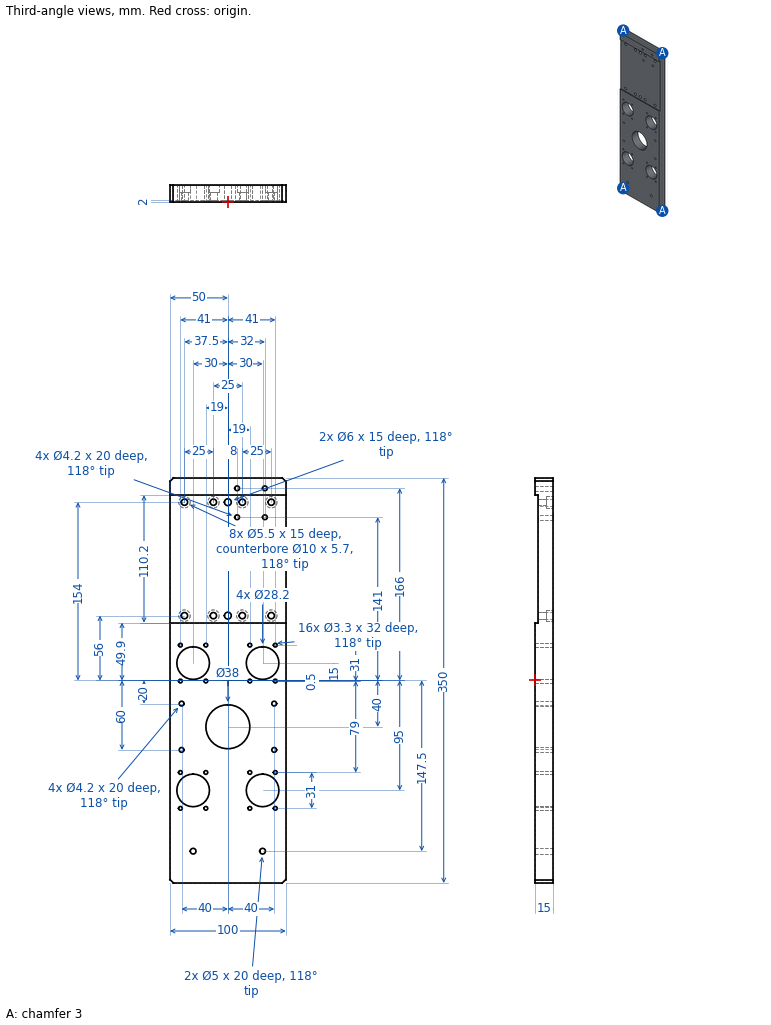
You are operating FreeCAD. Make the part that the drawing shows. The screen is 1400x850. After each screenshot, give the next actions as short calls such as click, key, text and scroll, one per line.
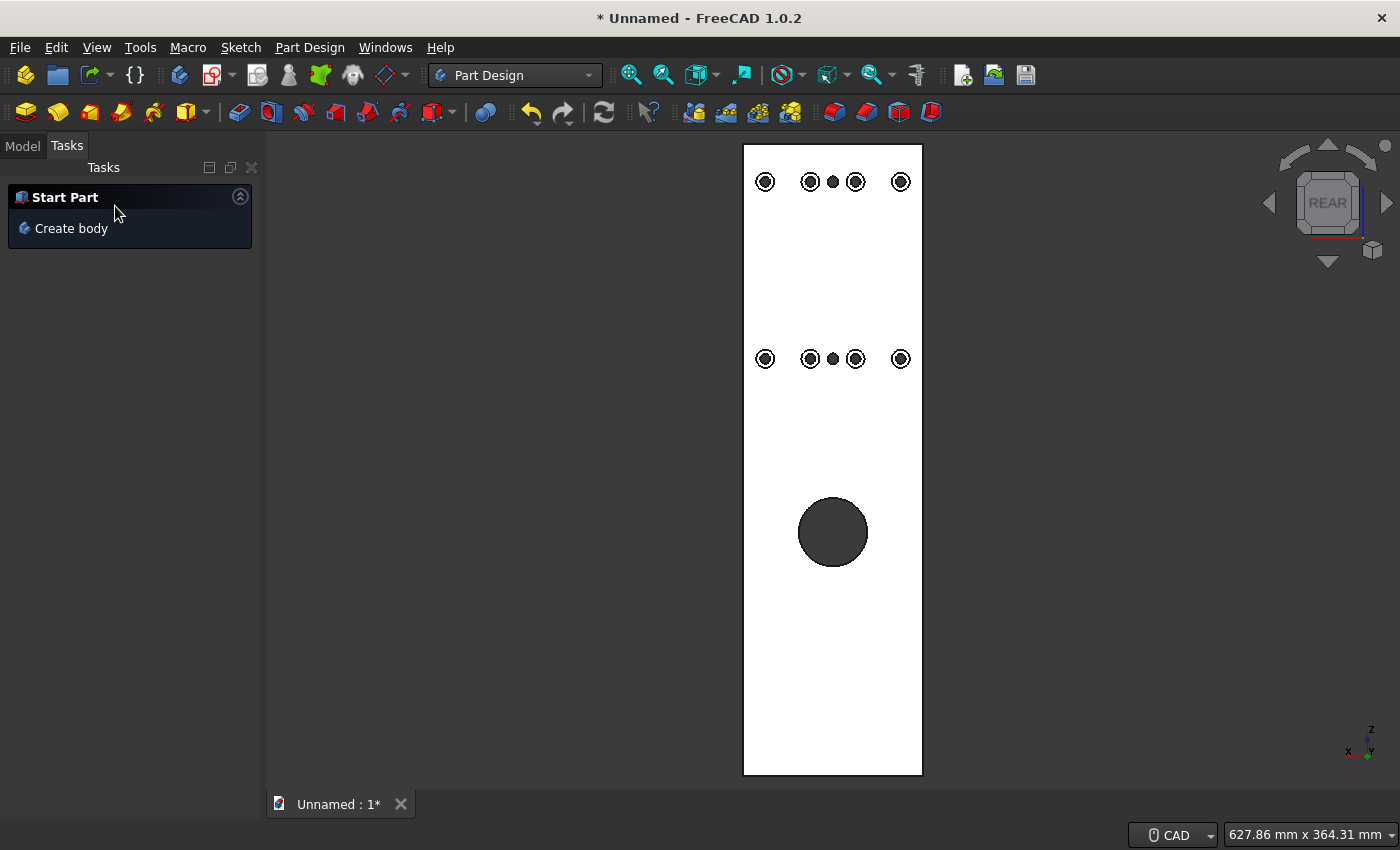
key(0)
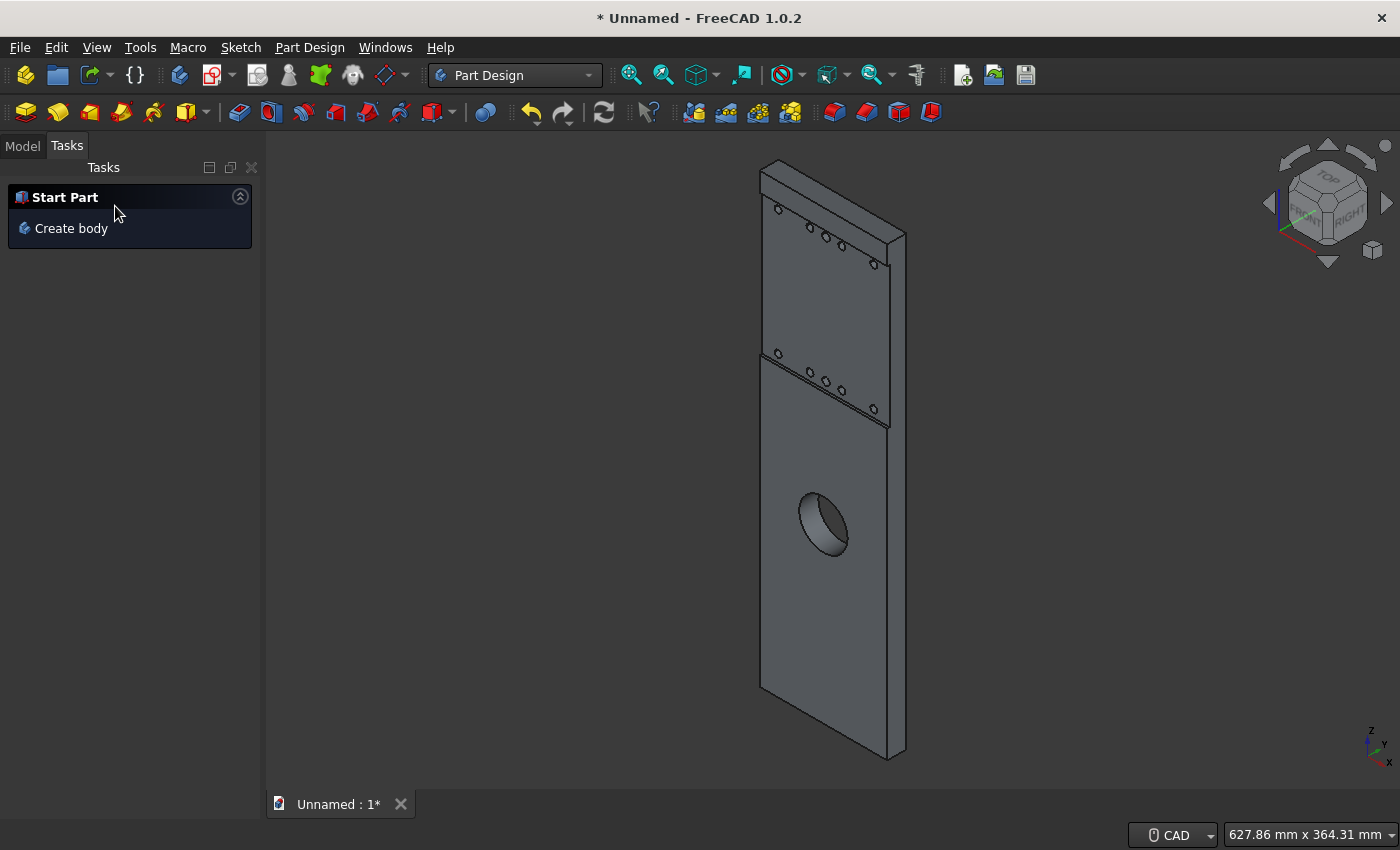
click(897, 238)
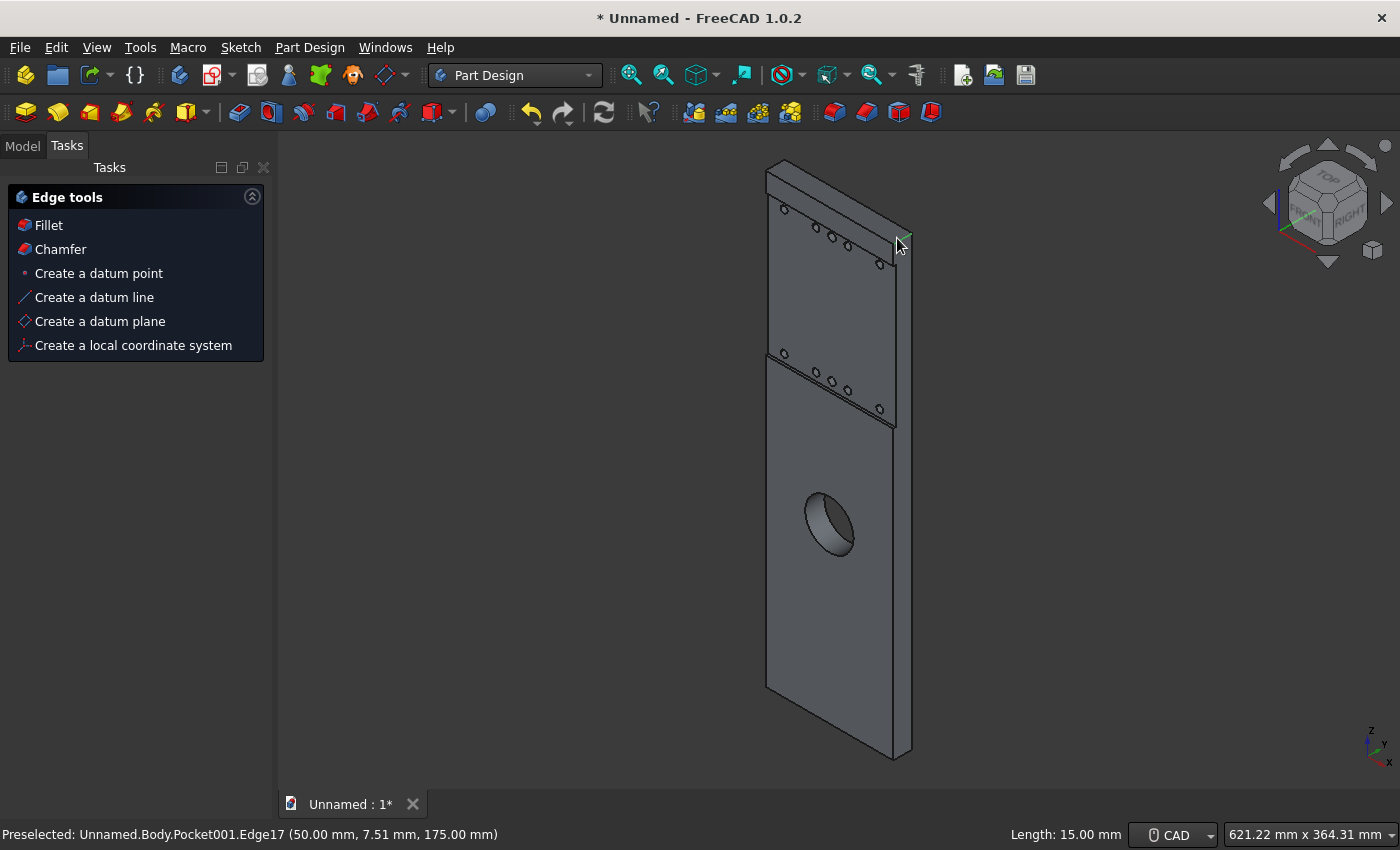
key(2)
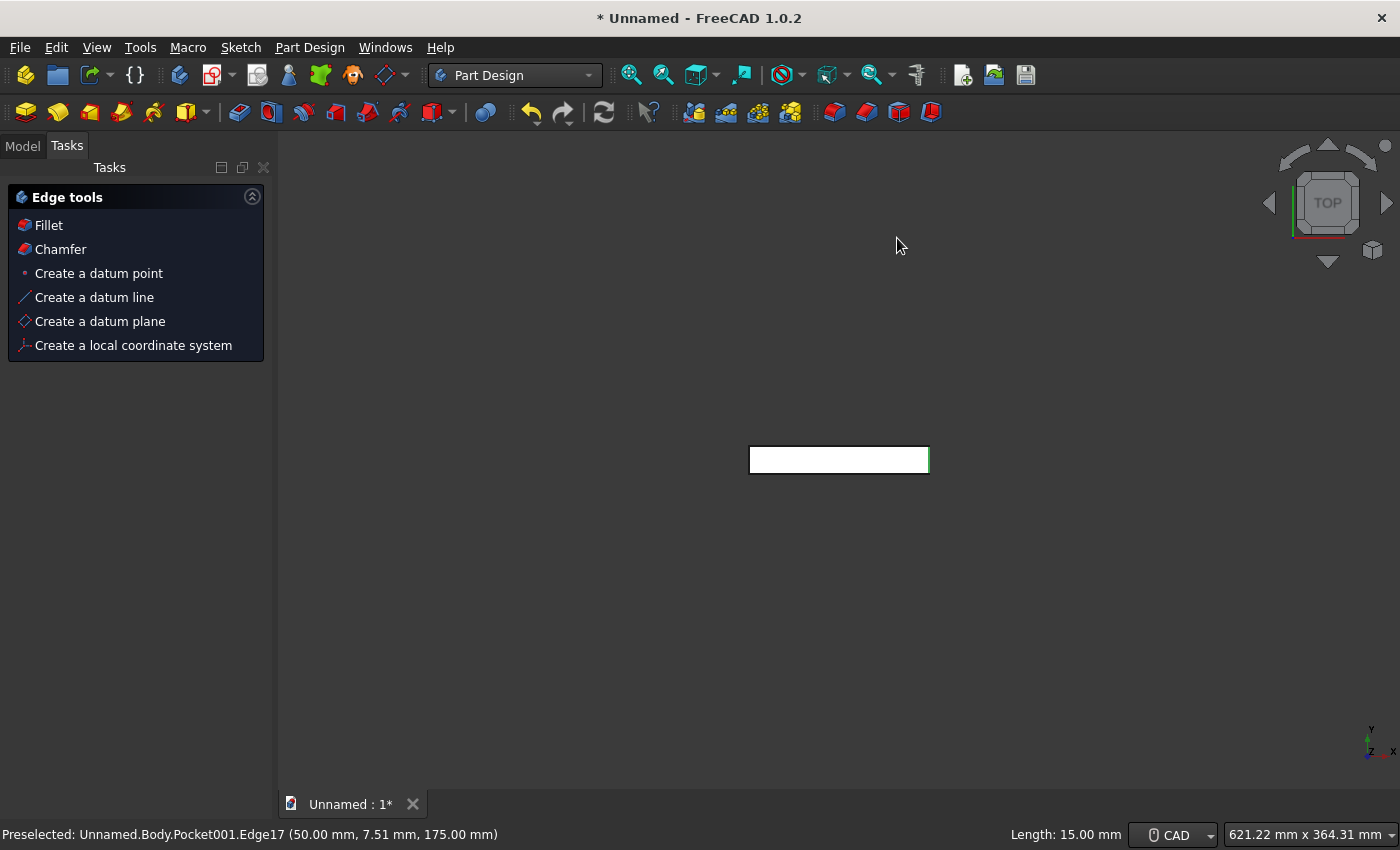
click(632, 76)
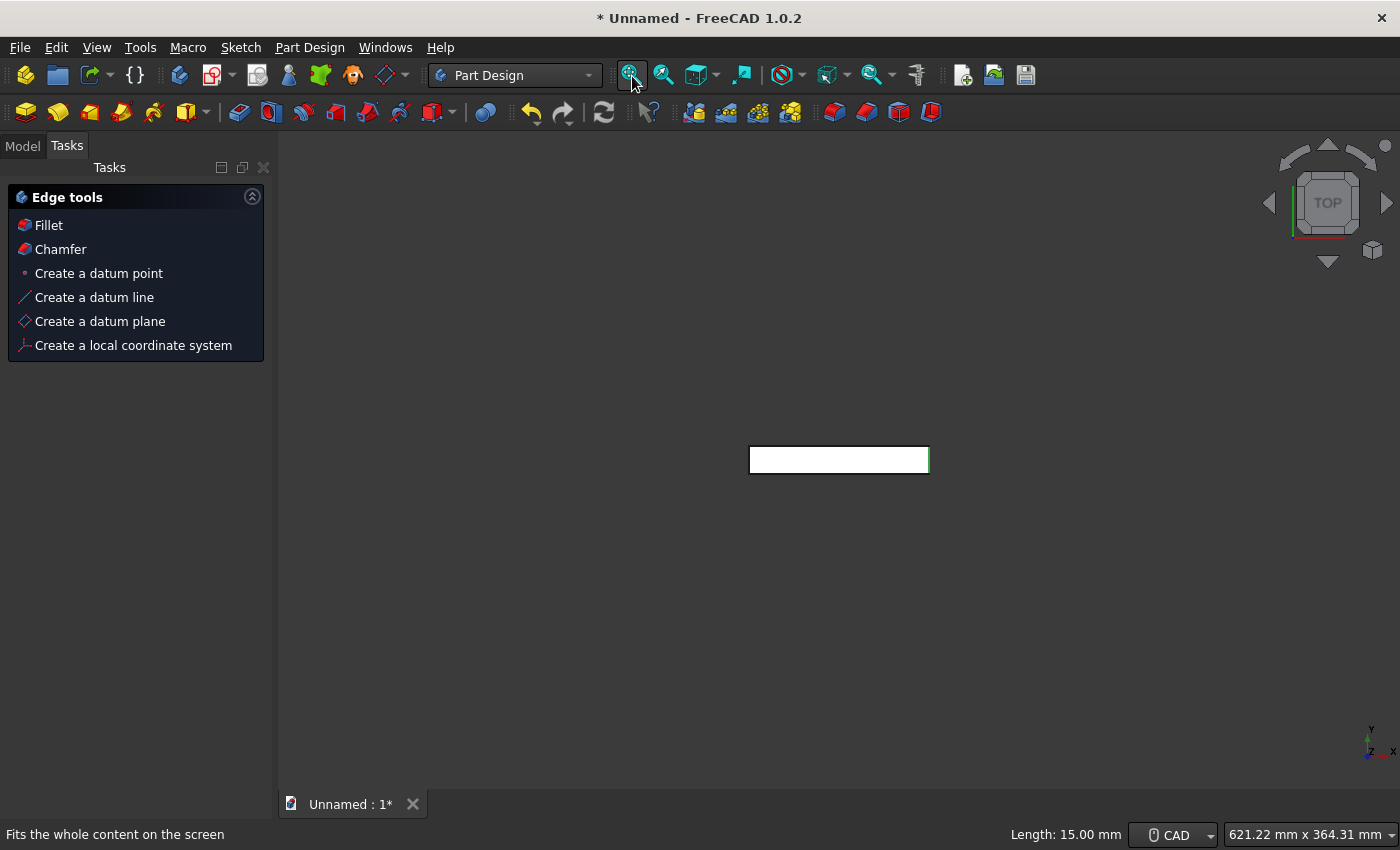
click(749, 459, ctrl)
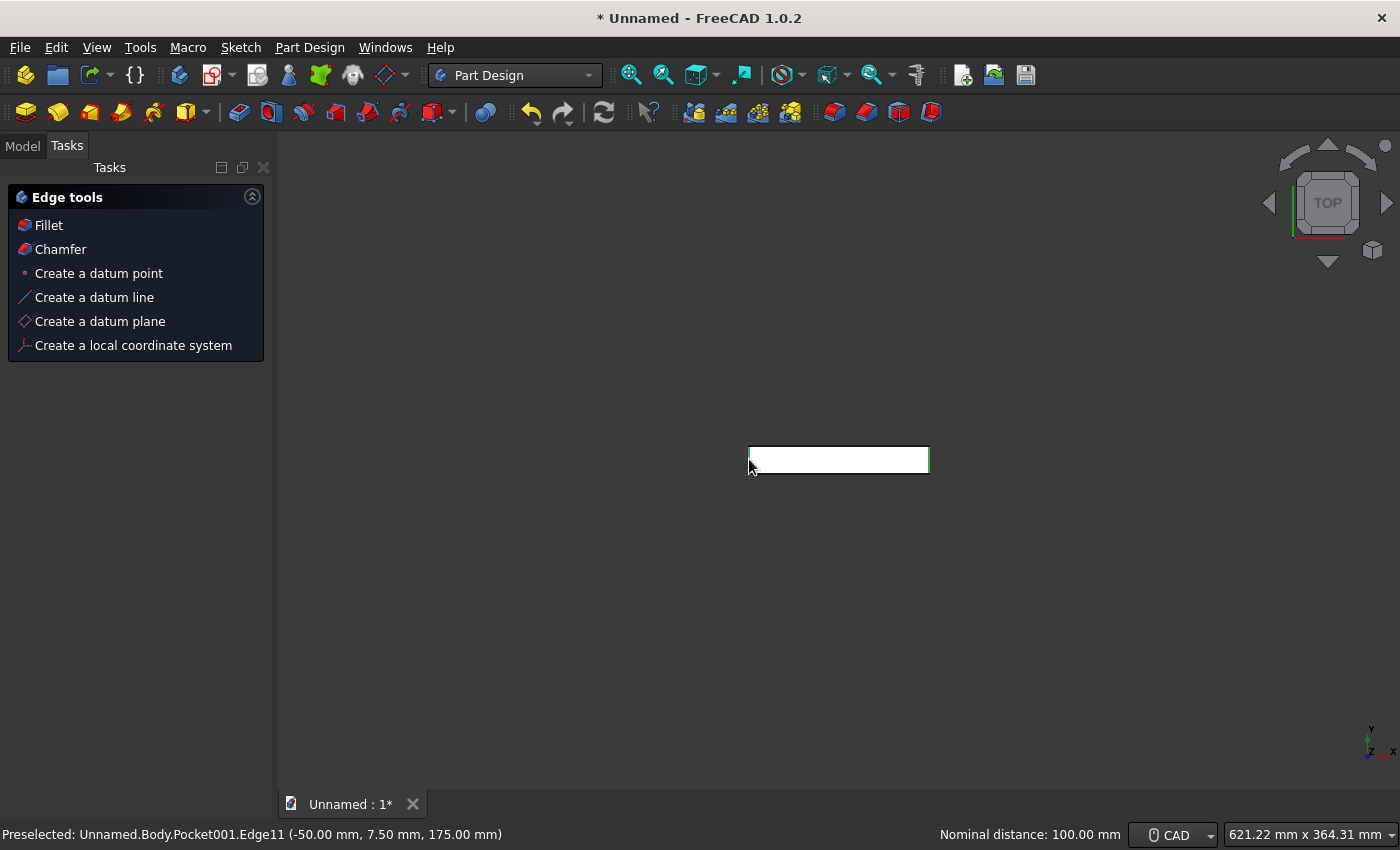
key(1)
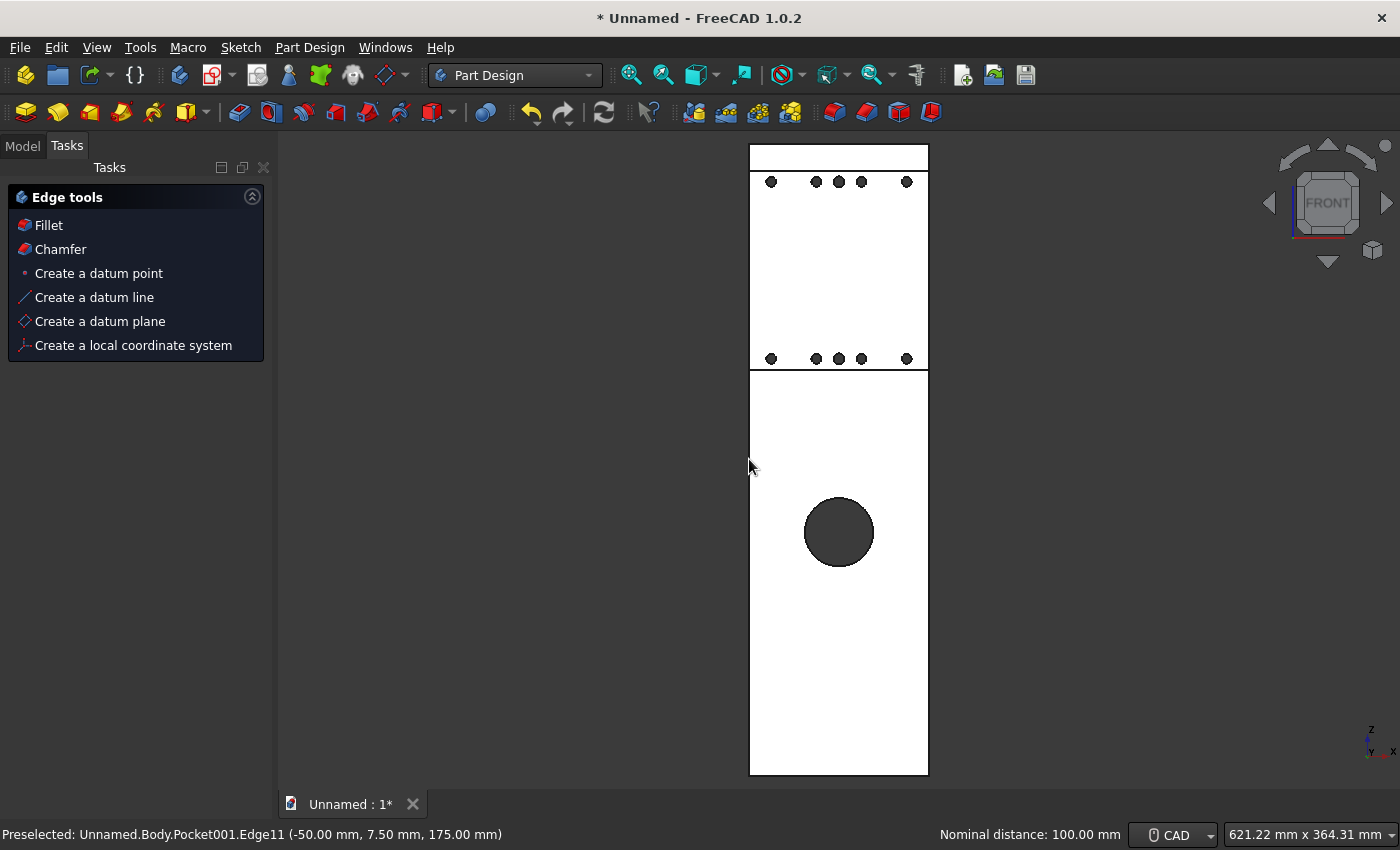
key(3)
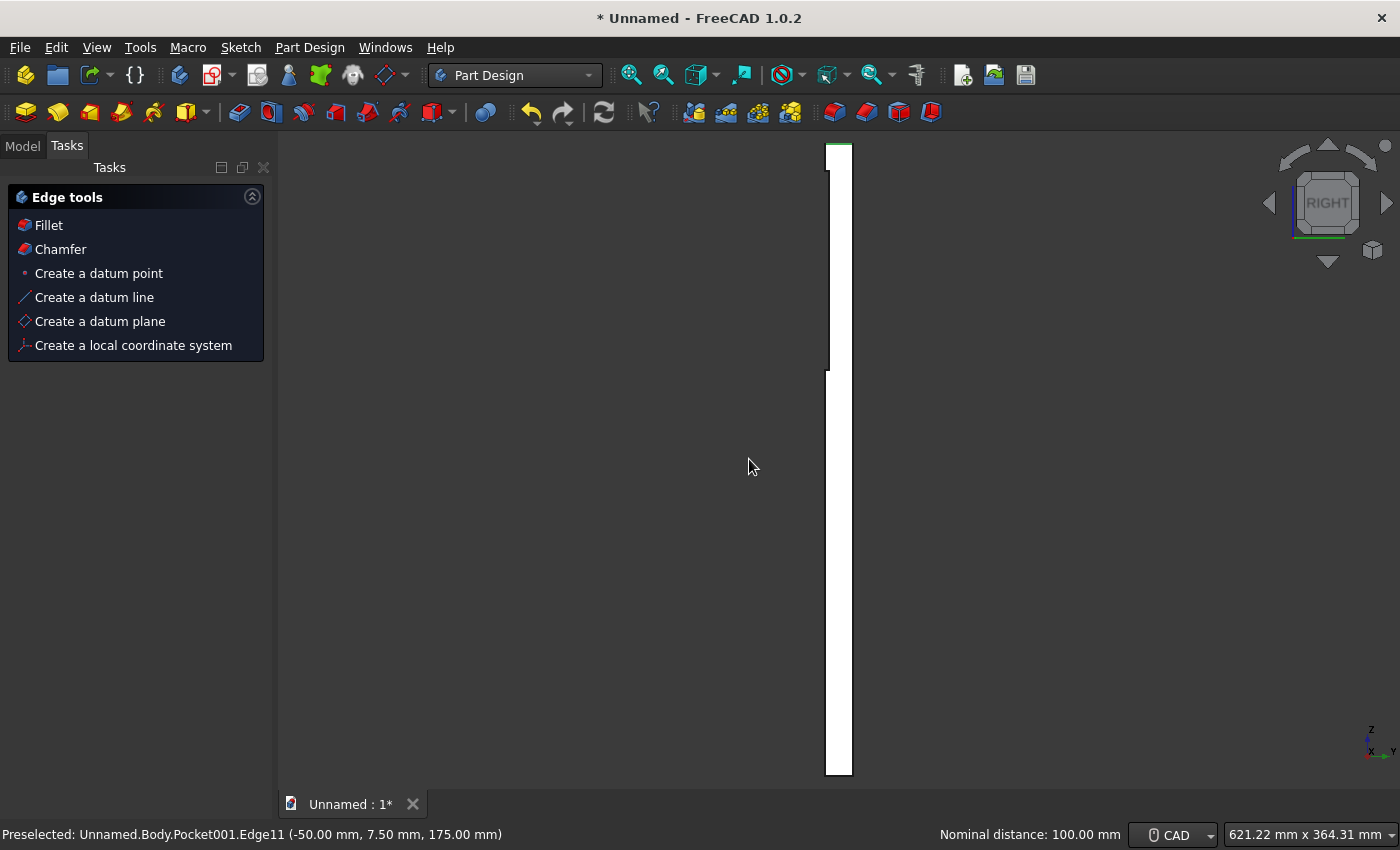
key(5)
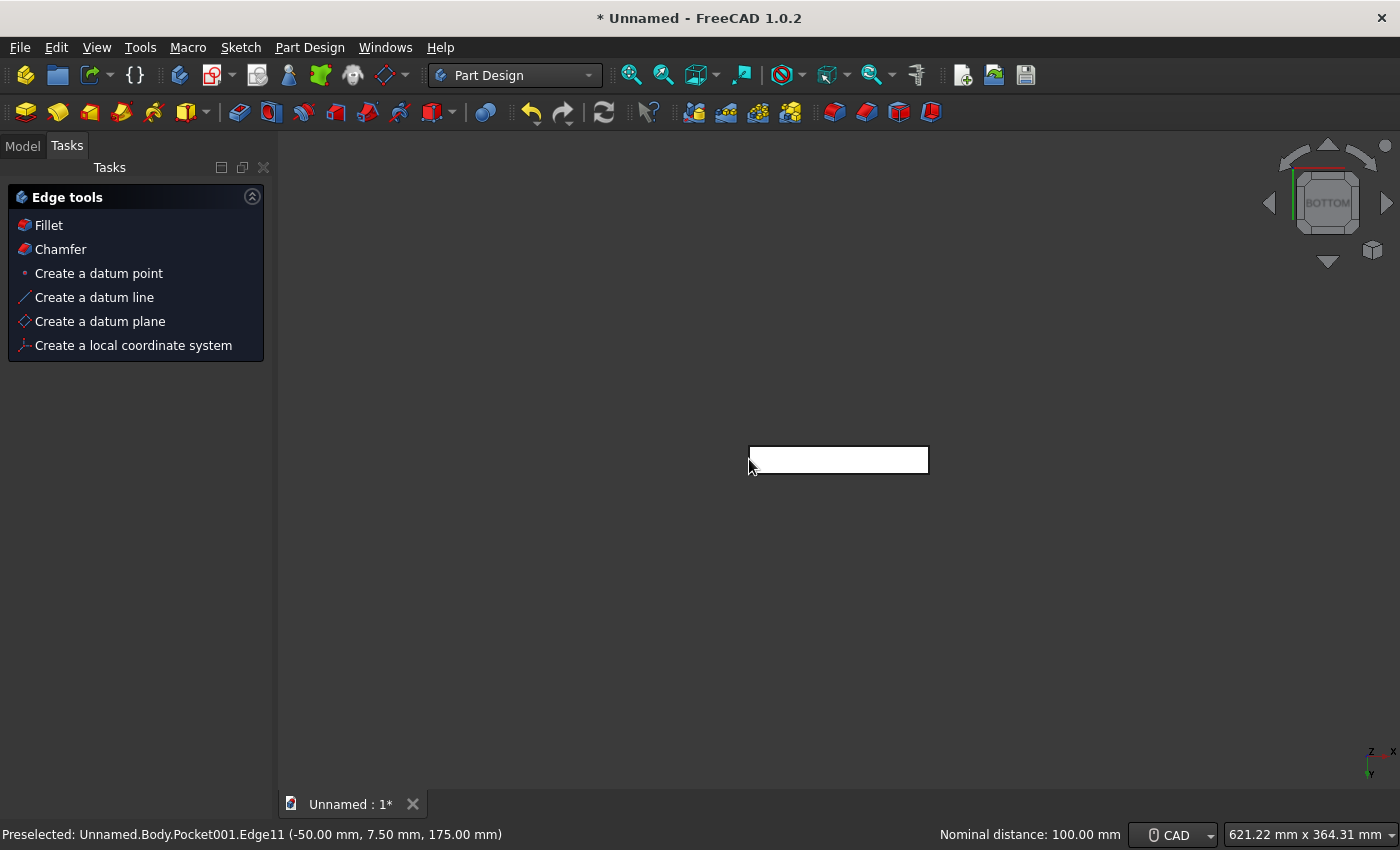
click(632, 76)